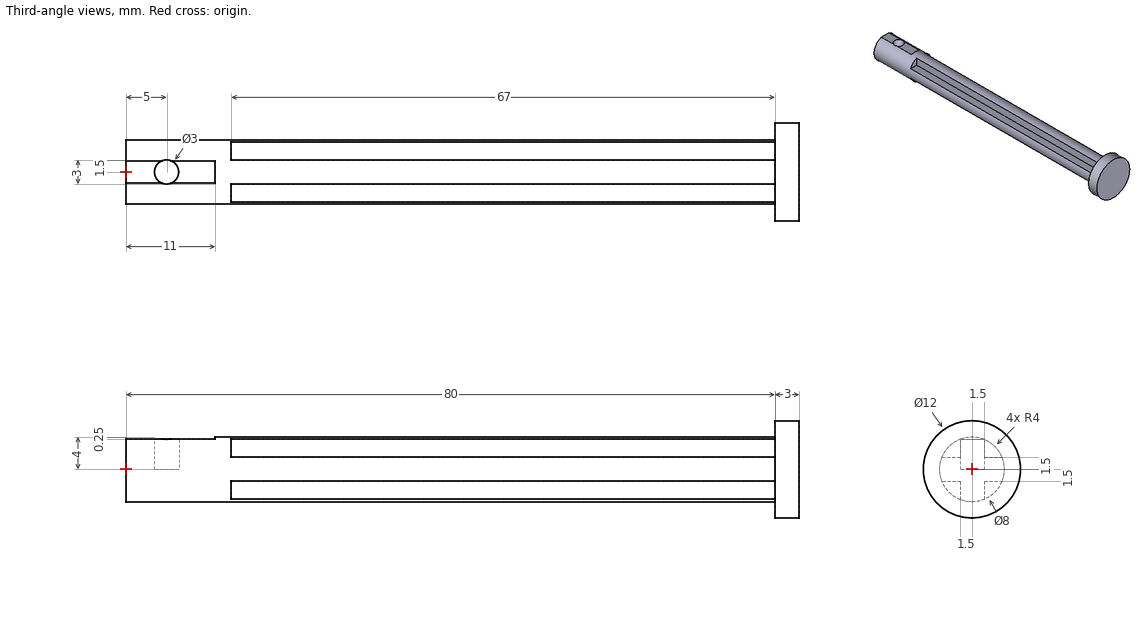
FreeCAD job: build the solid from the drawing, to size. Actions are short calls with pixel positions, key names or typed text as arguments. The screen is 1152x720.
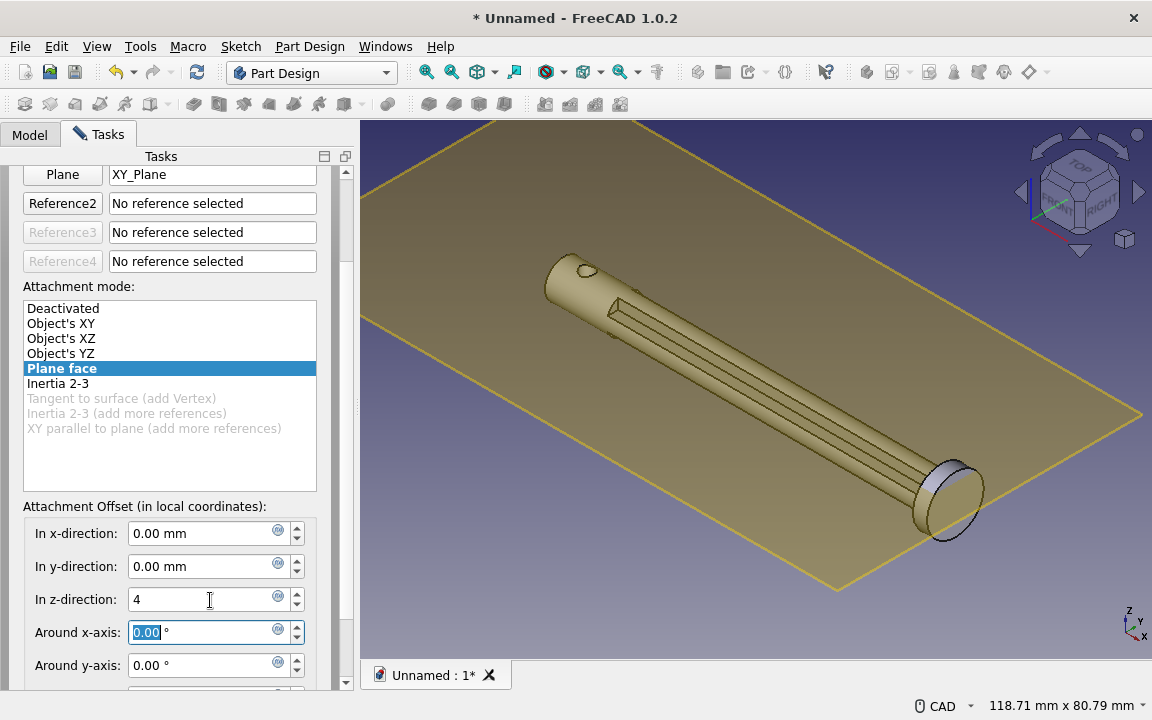
scroll(346, 428, up, 3)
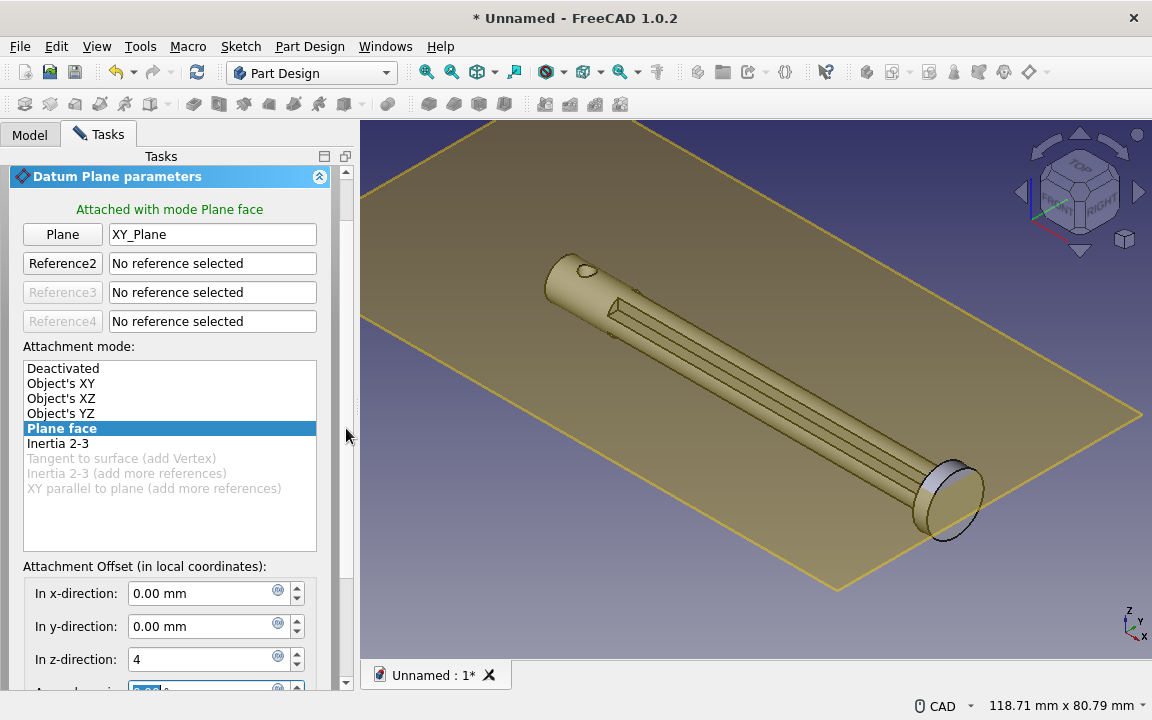
click(127, 195)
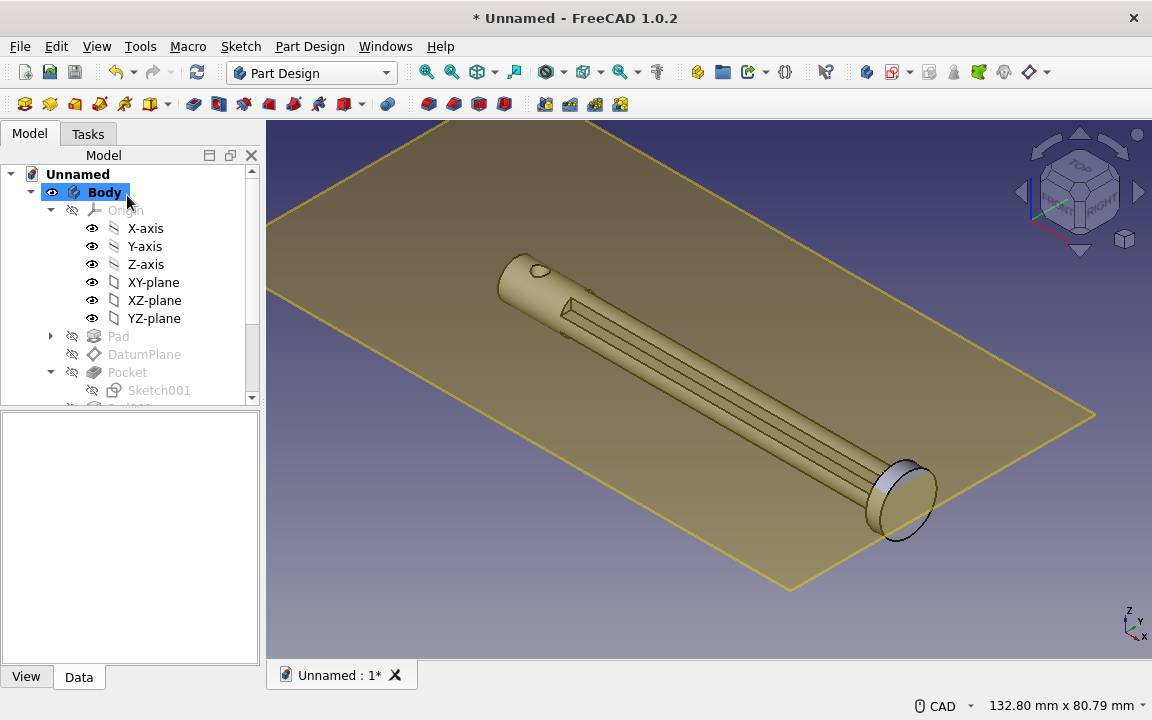
scroll(101, 278, down, 3)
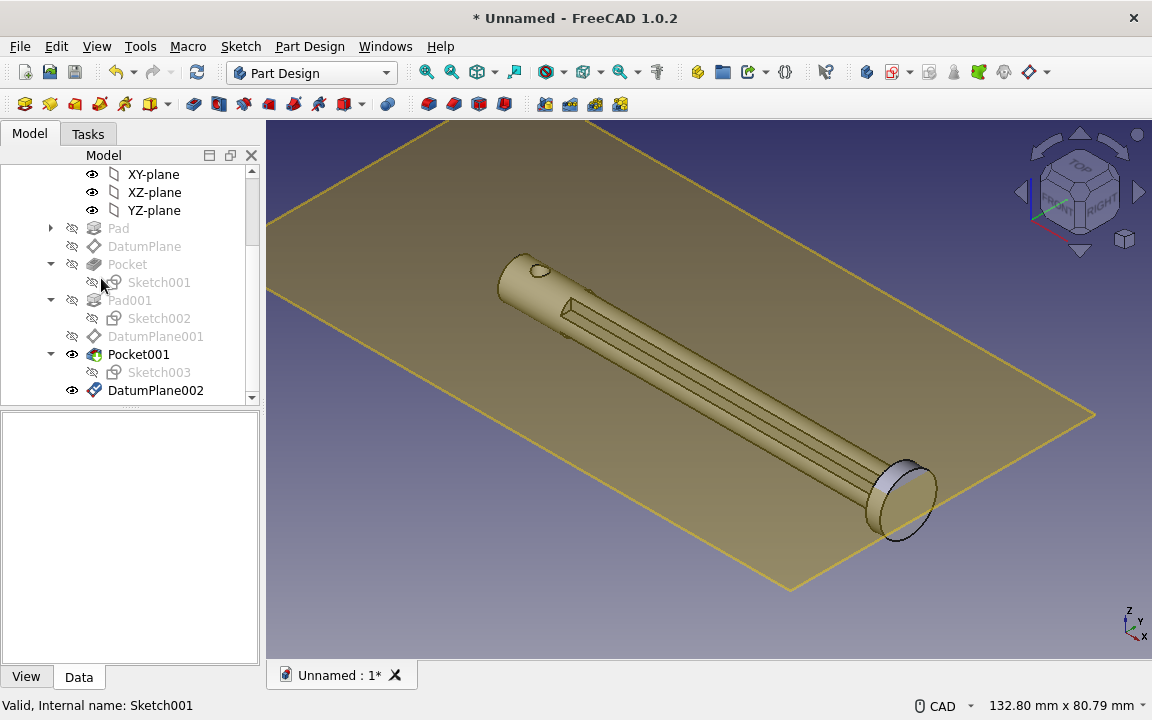
click(117, 390)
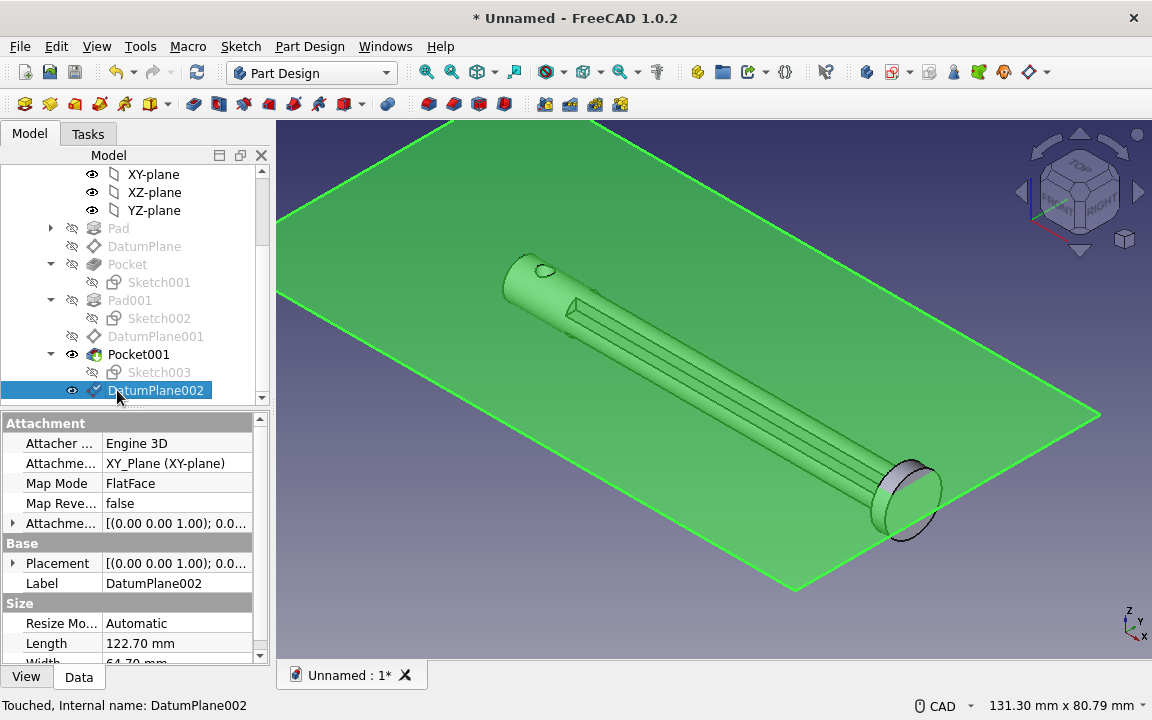
click(892, 72)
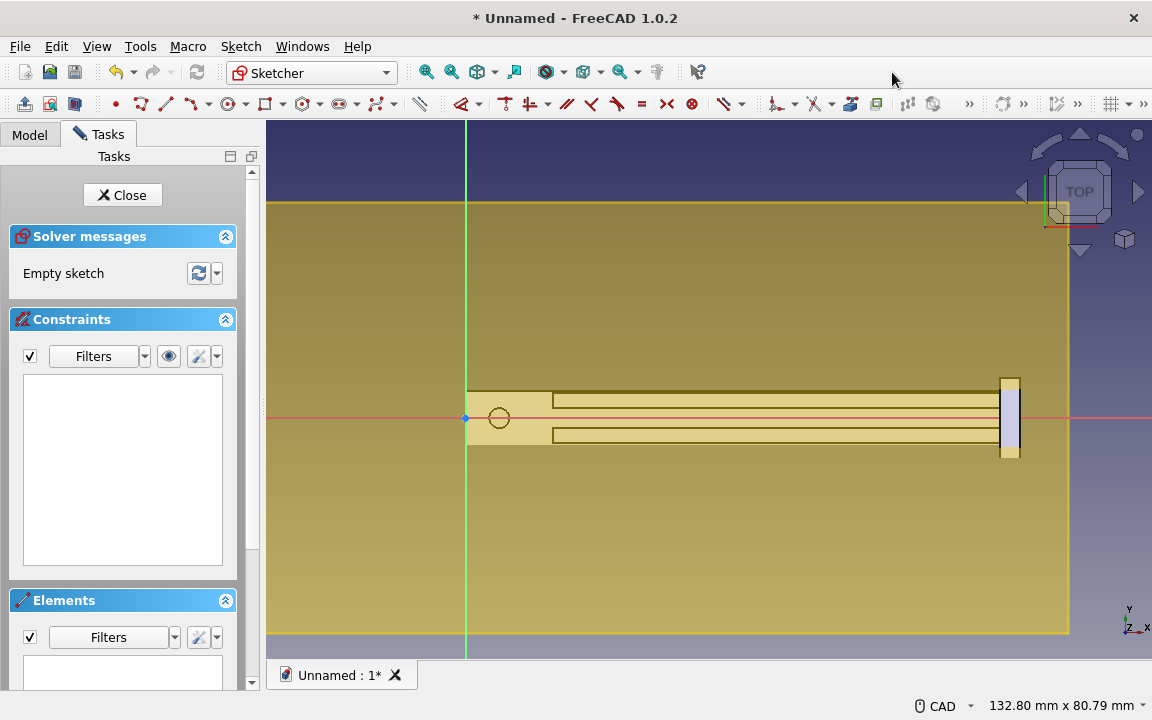
key(q)
key(s)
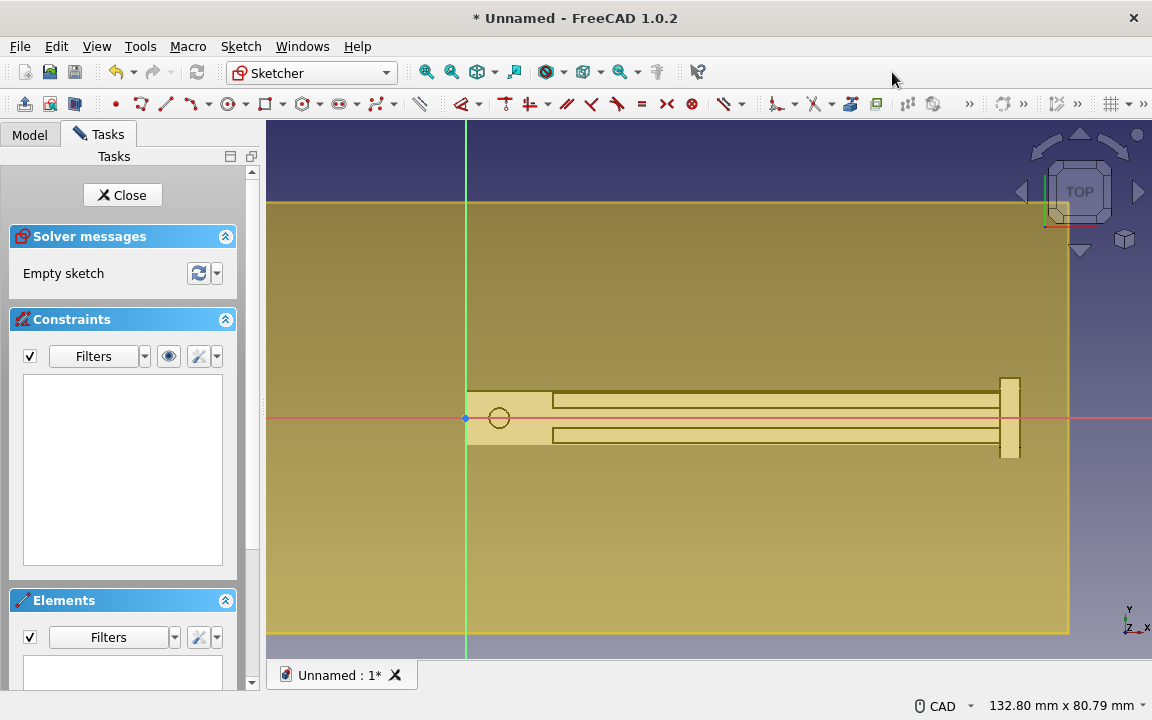
scroll(475, 424, up, 9)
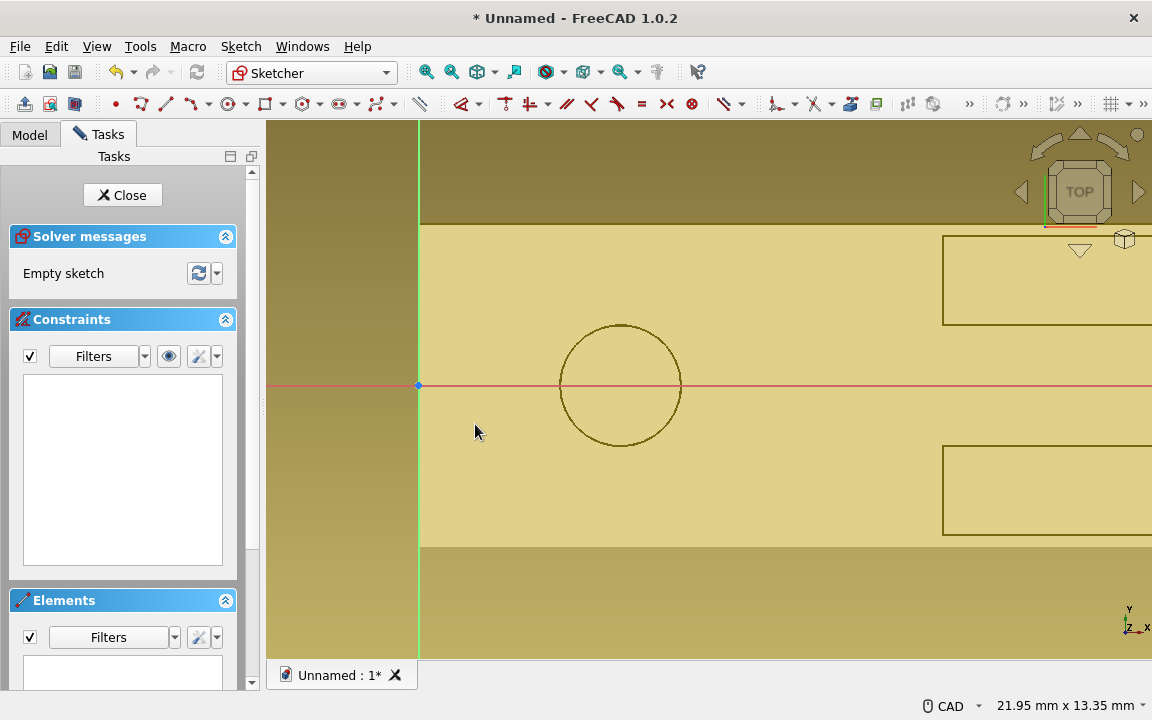
click(264, 104)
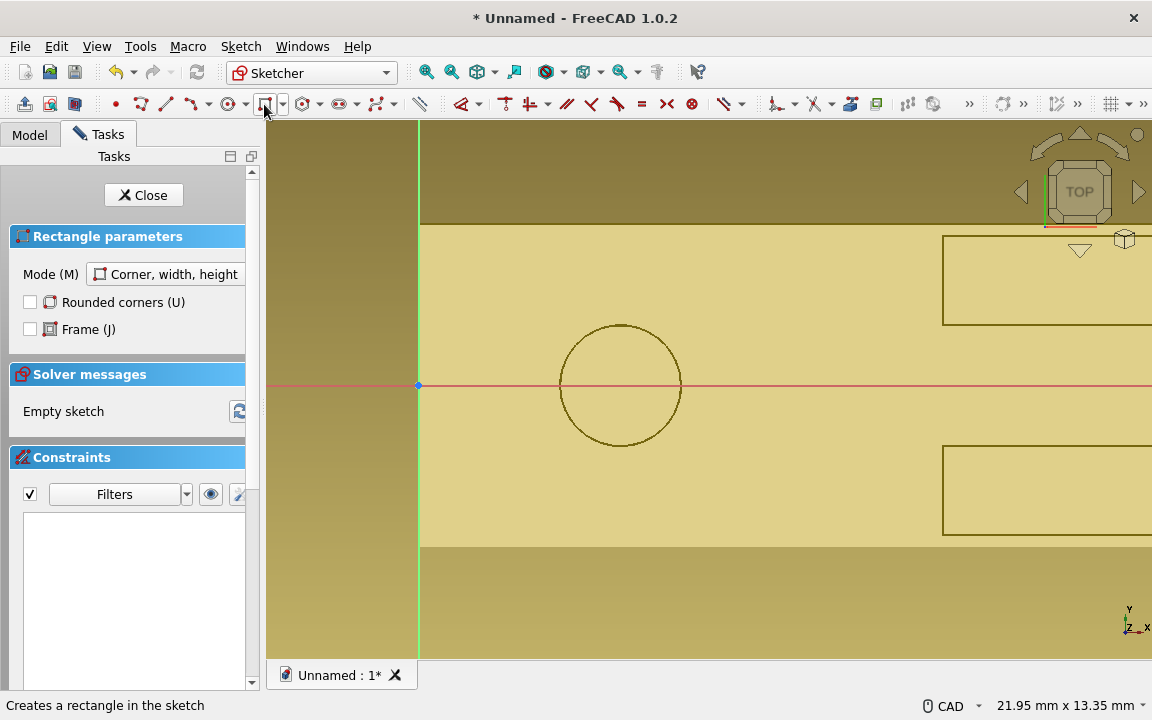
click(419, 325)
move(863, 446)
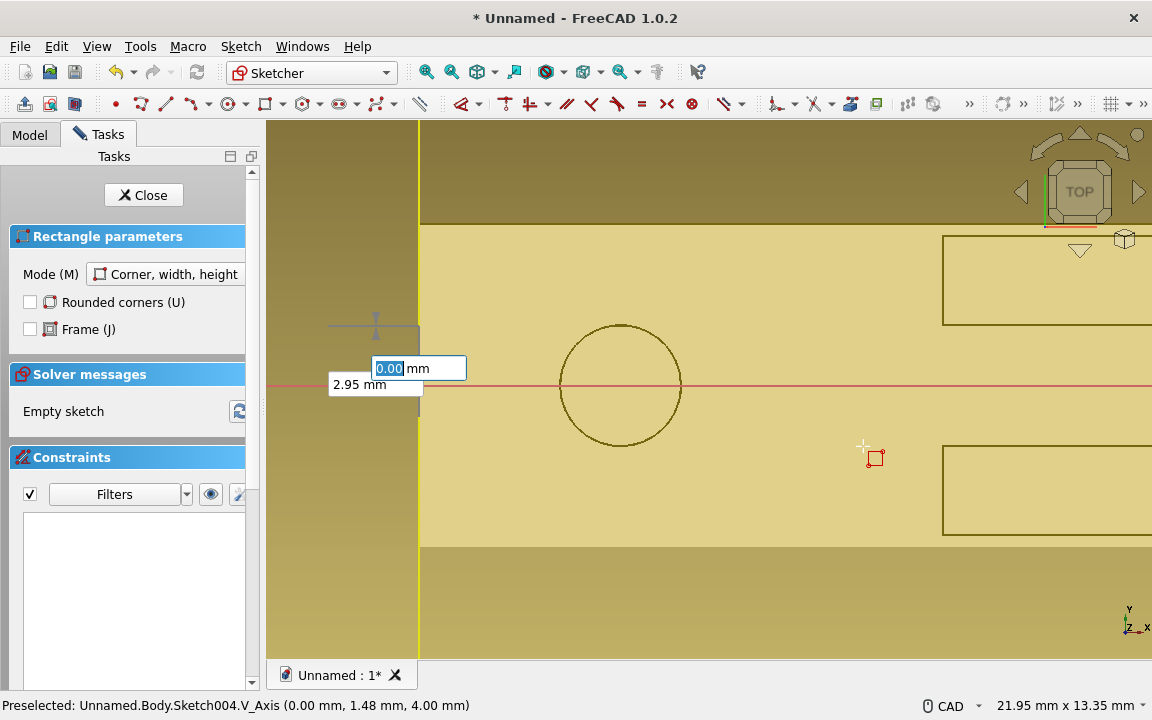
text(11)
key(Tab)
text(3)
key(Return)
key(Escape)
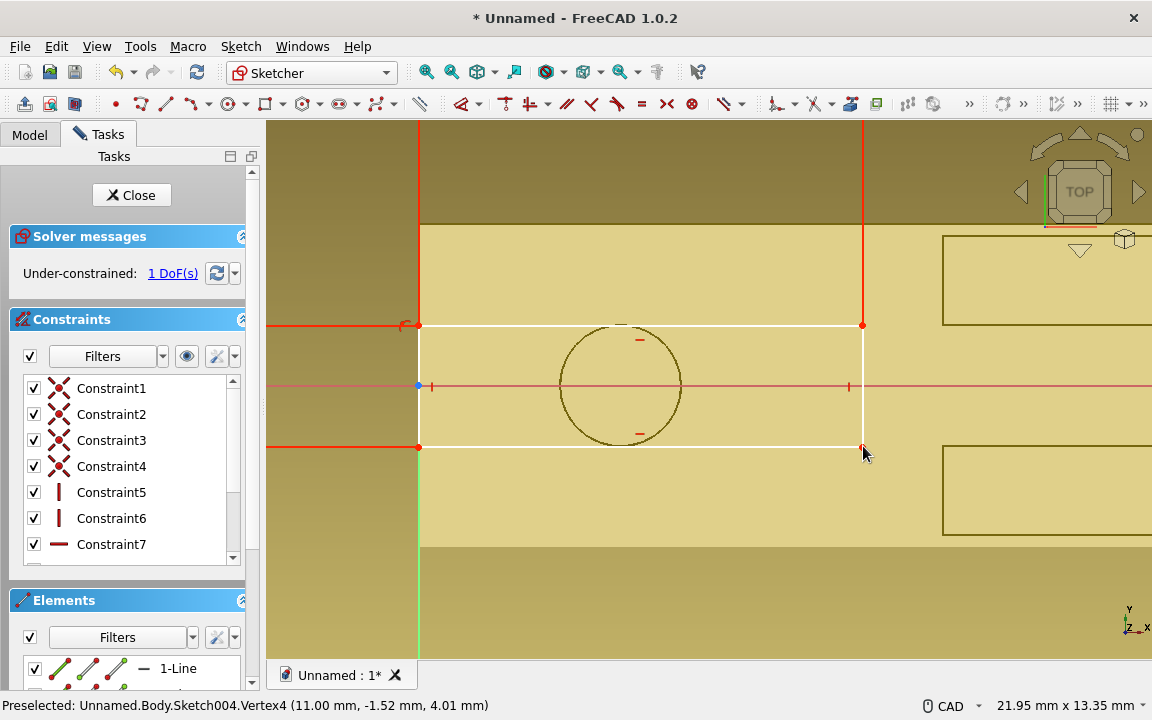
click(419, 326)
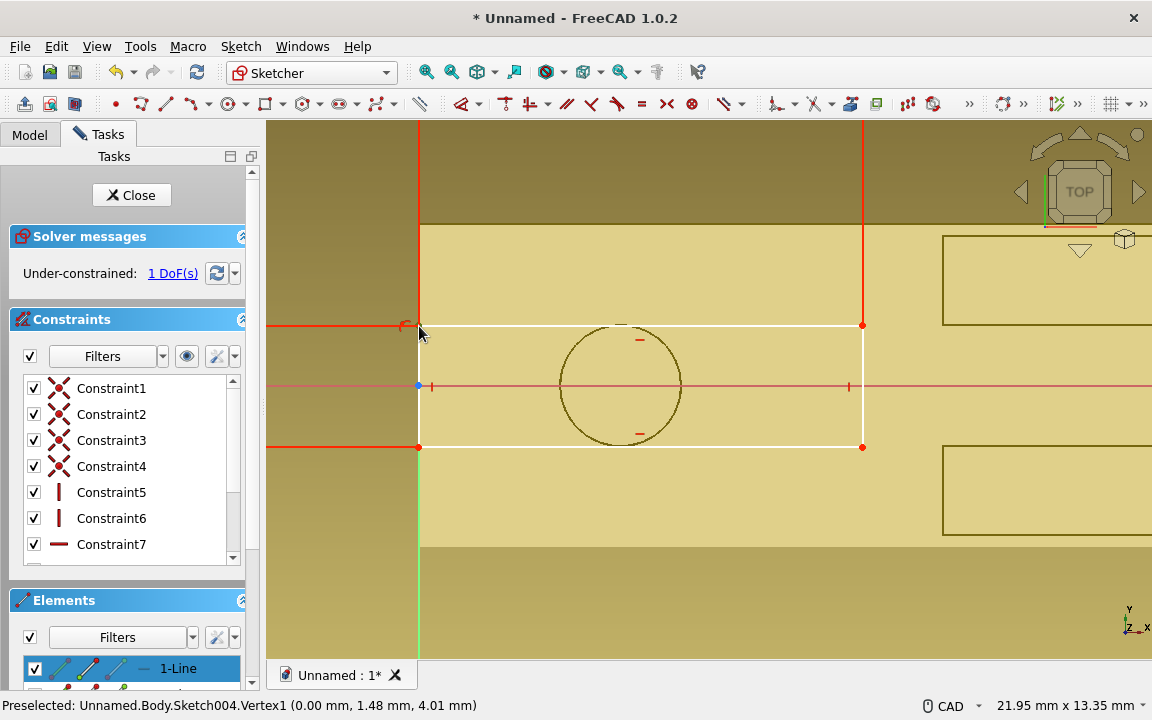
key(i)